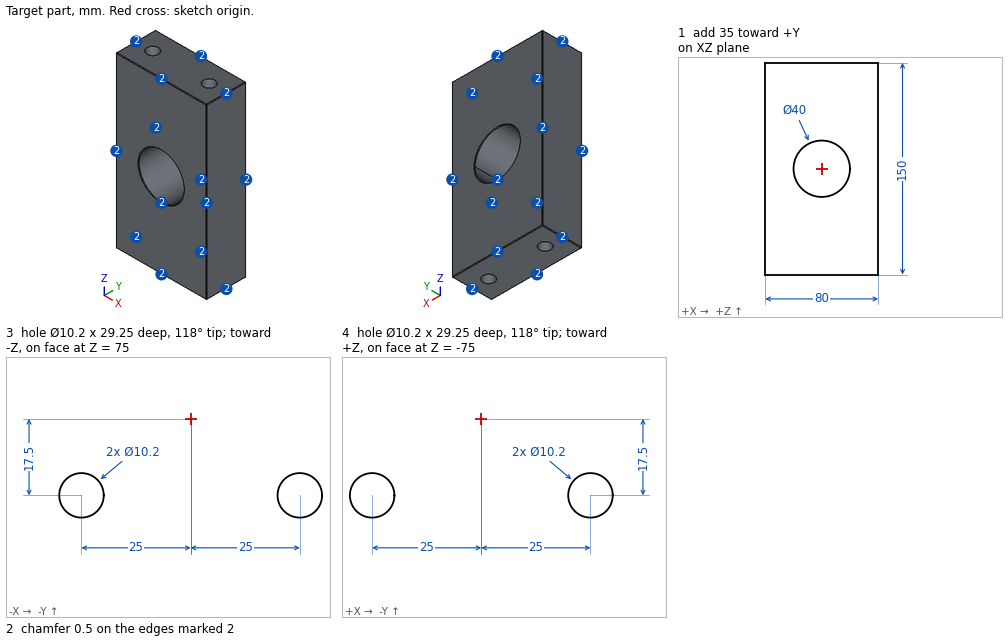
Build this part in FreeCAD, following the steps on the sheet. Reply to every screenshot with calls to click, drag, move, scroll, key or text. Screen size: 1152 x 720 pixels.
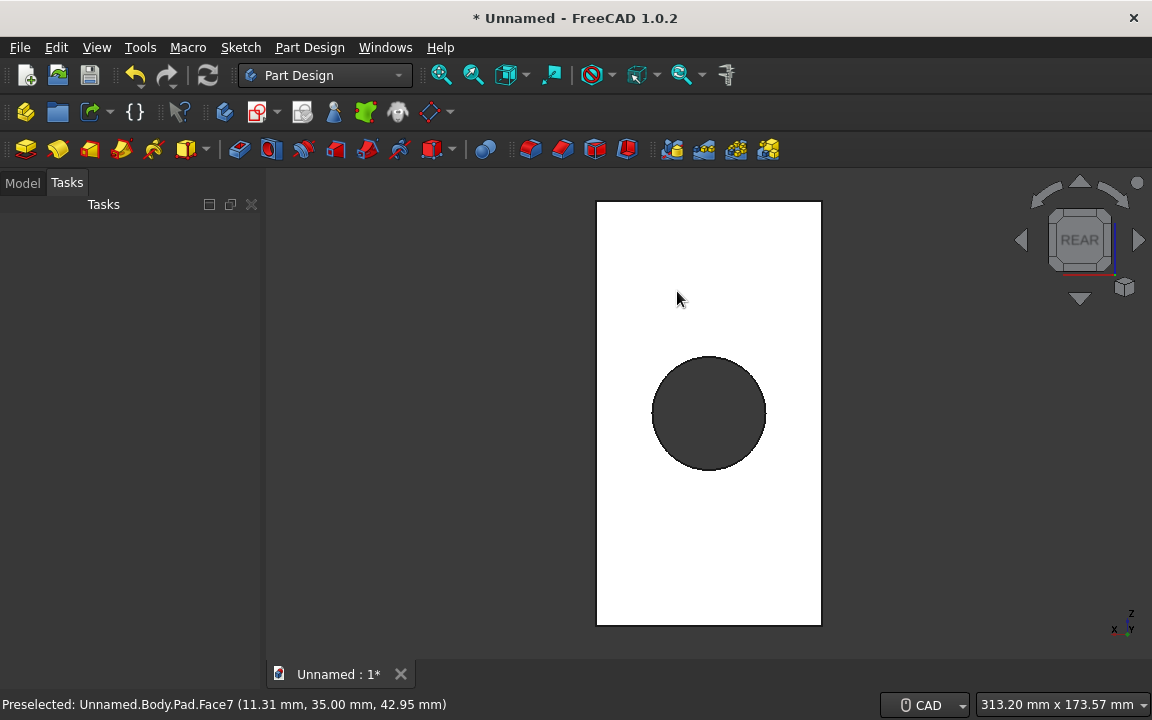
click(564, 150)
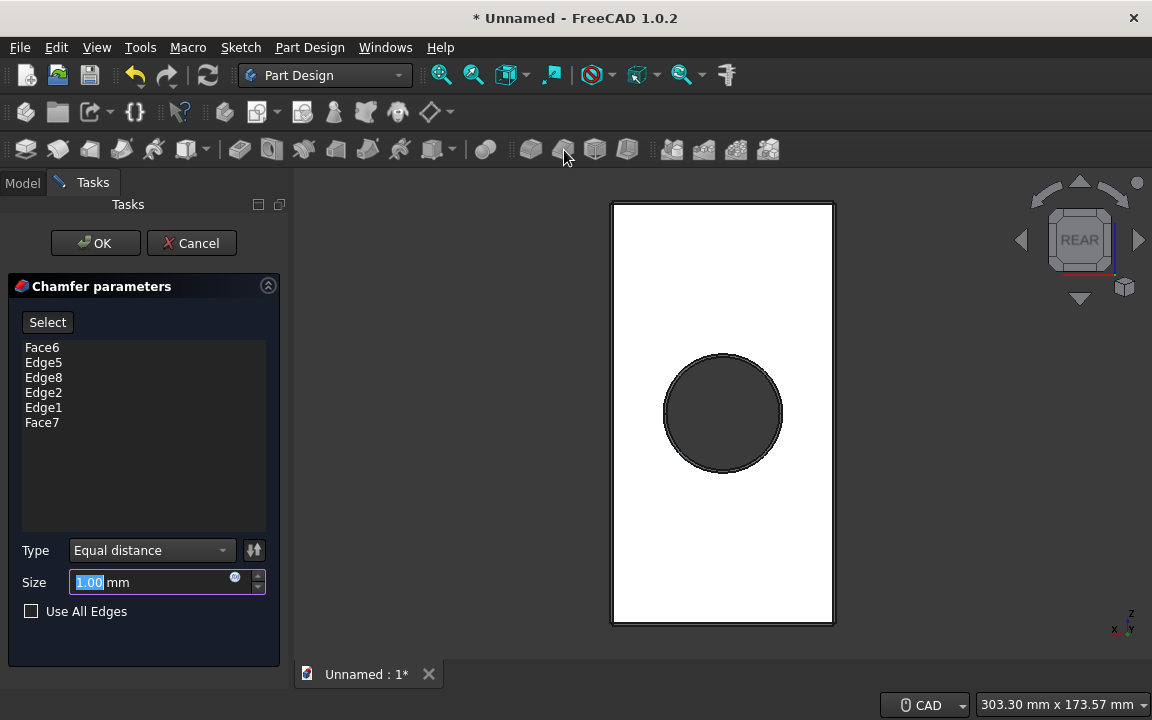
text(0.5)
key(Tab)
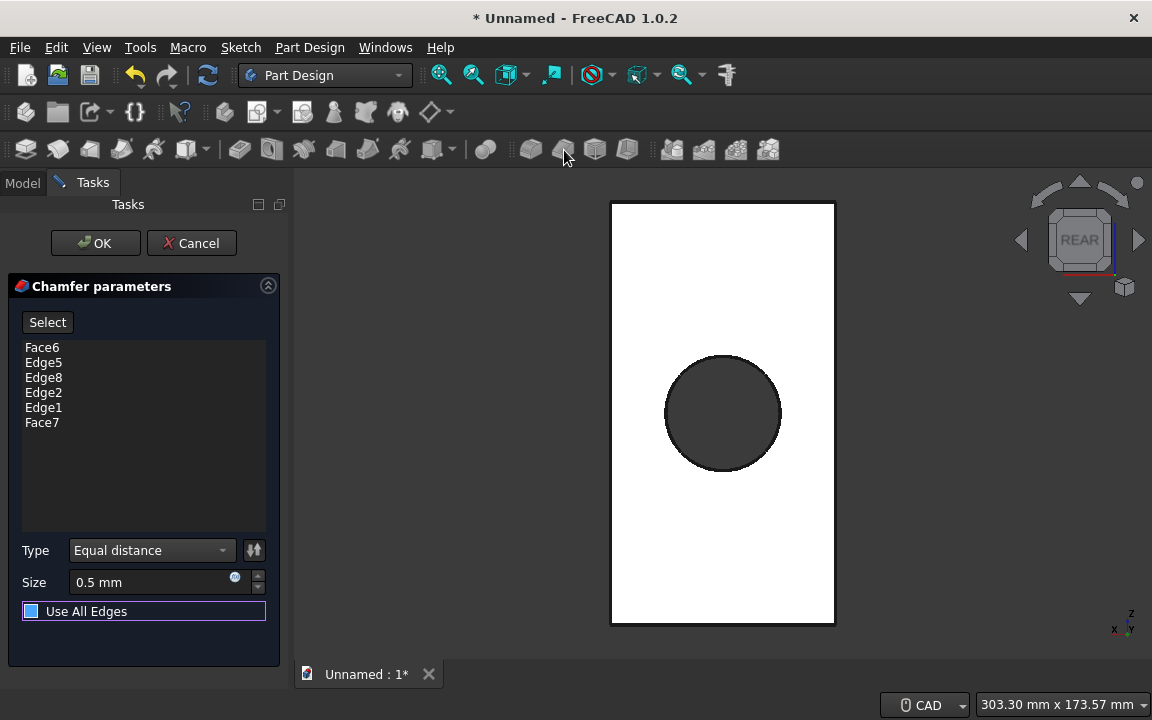
click(96, 243)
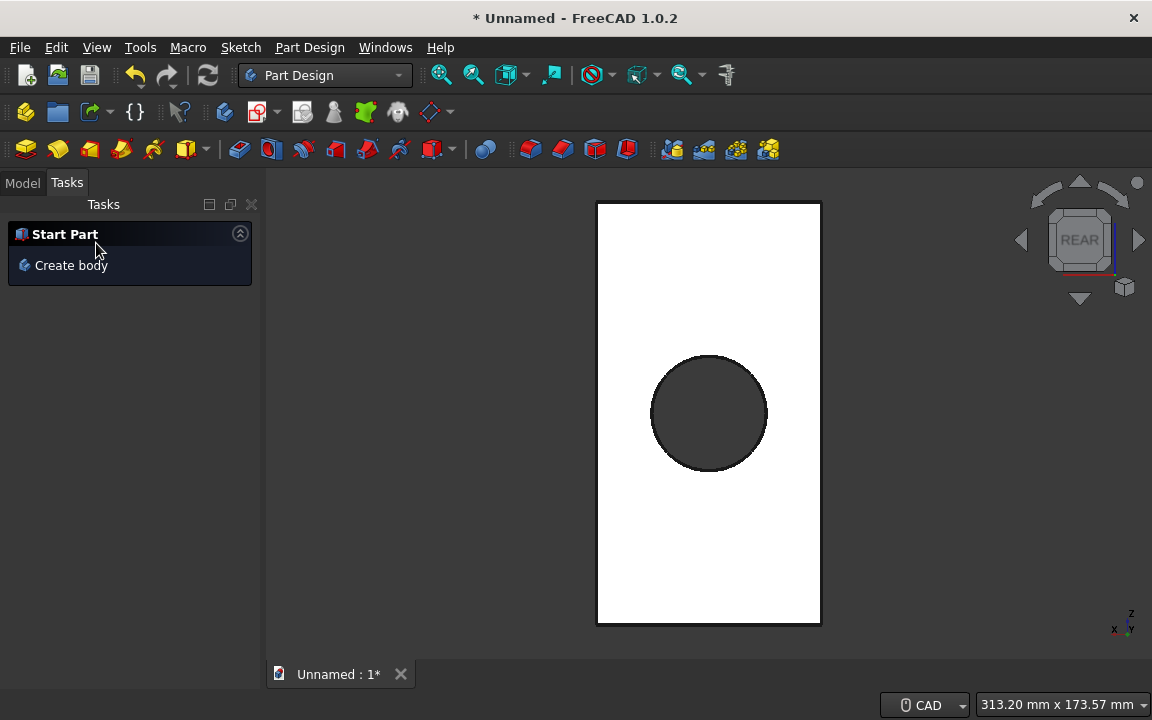
key(0)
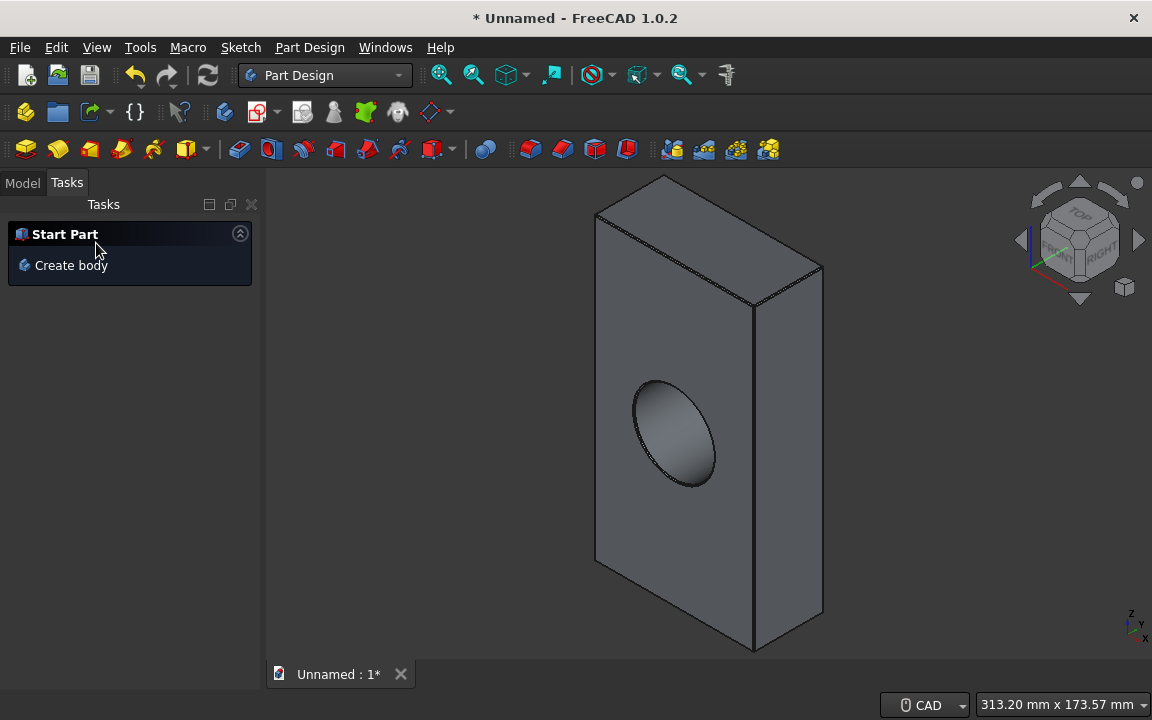
click(732, 252)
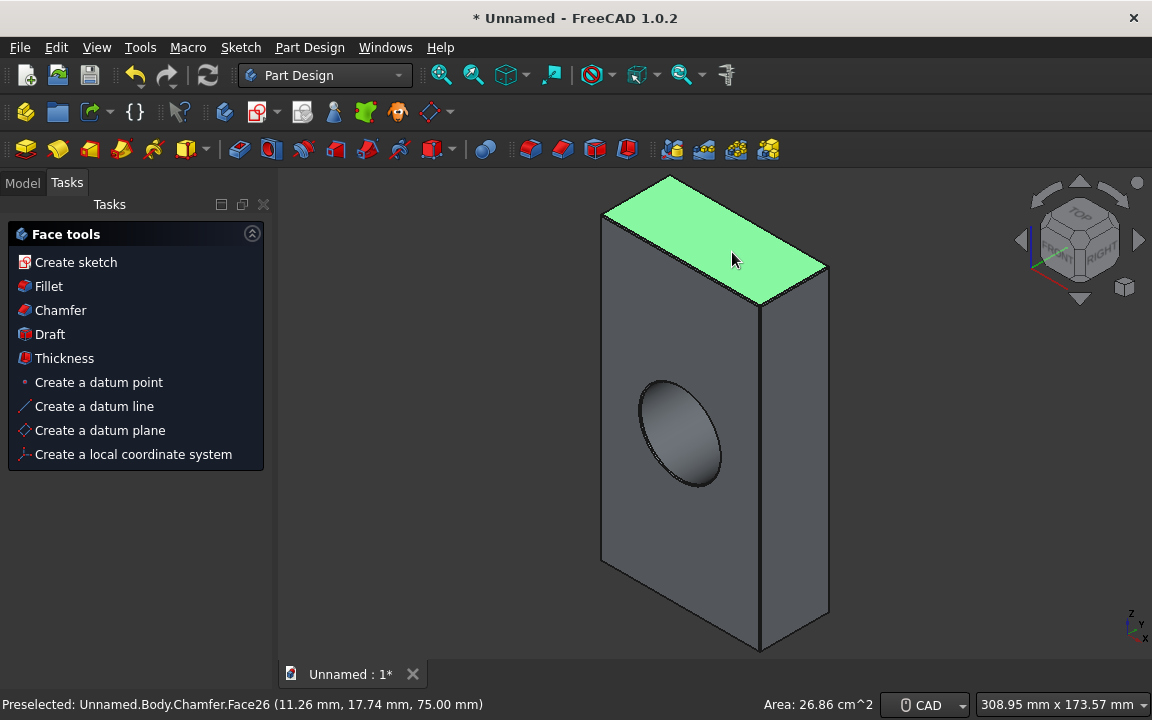
click(258, 112)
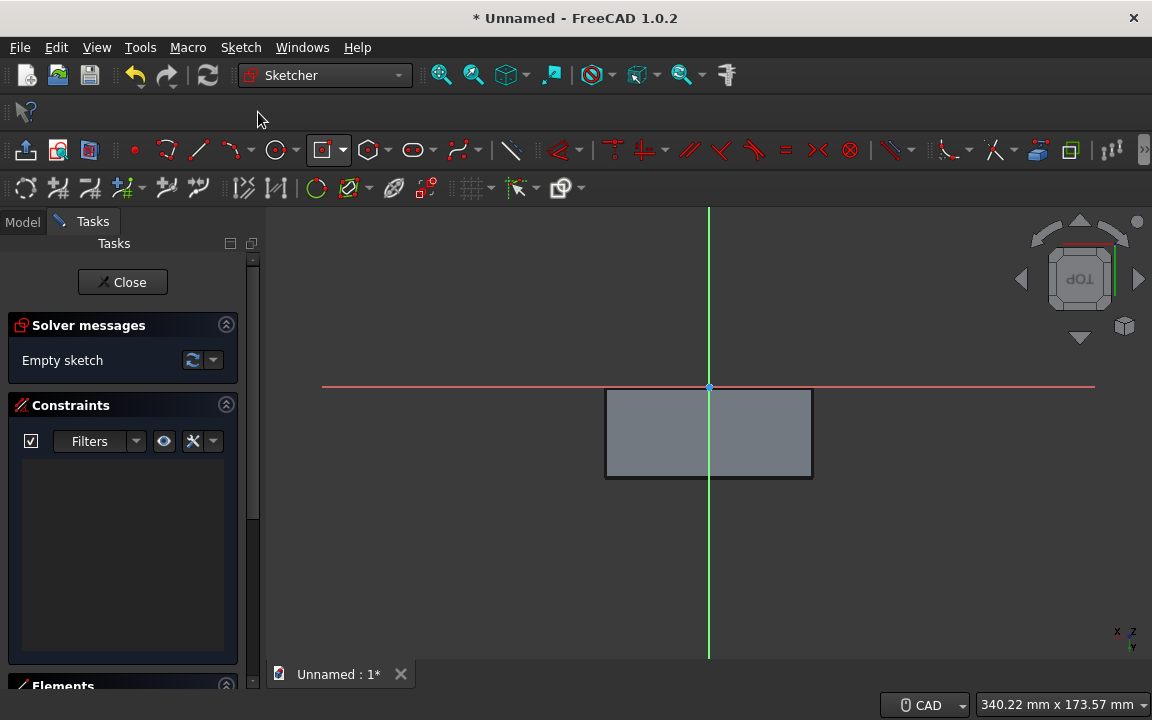
scroll(739, 410, up, 6)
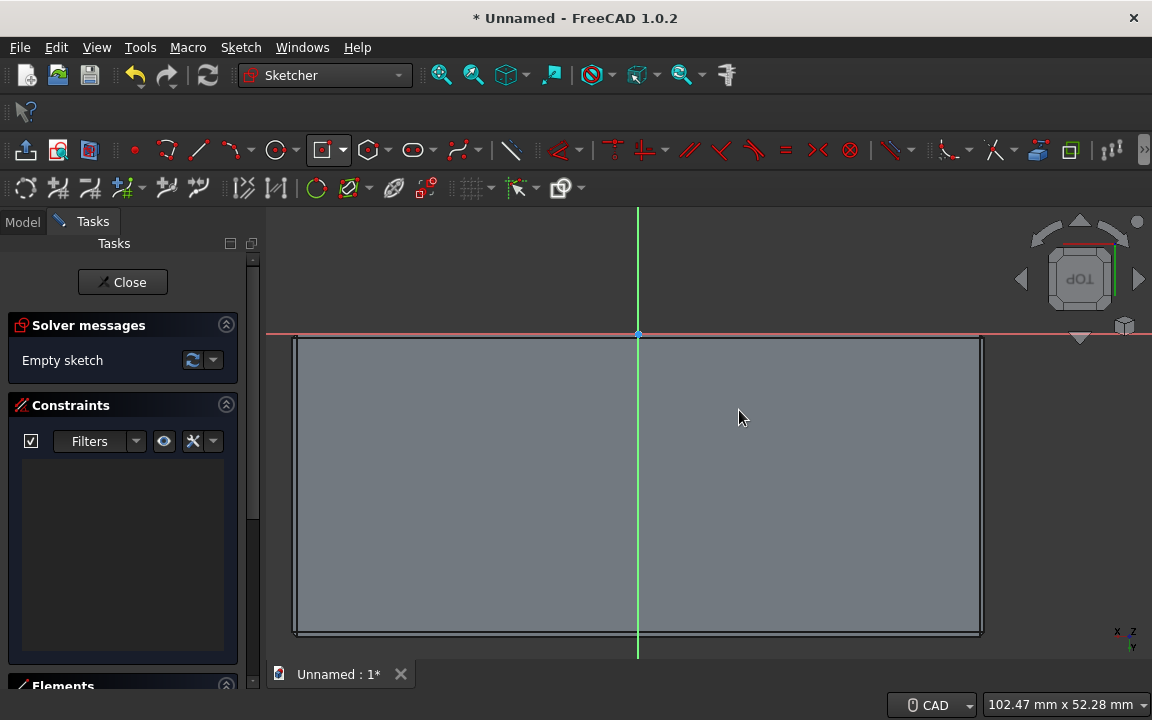
key(g)
key(c)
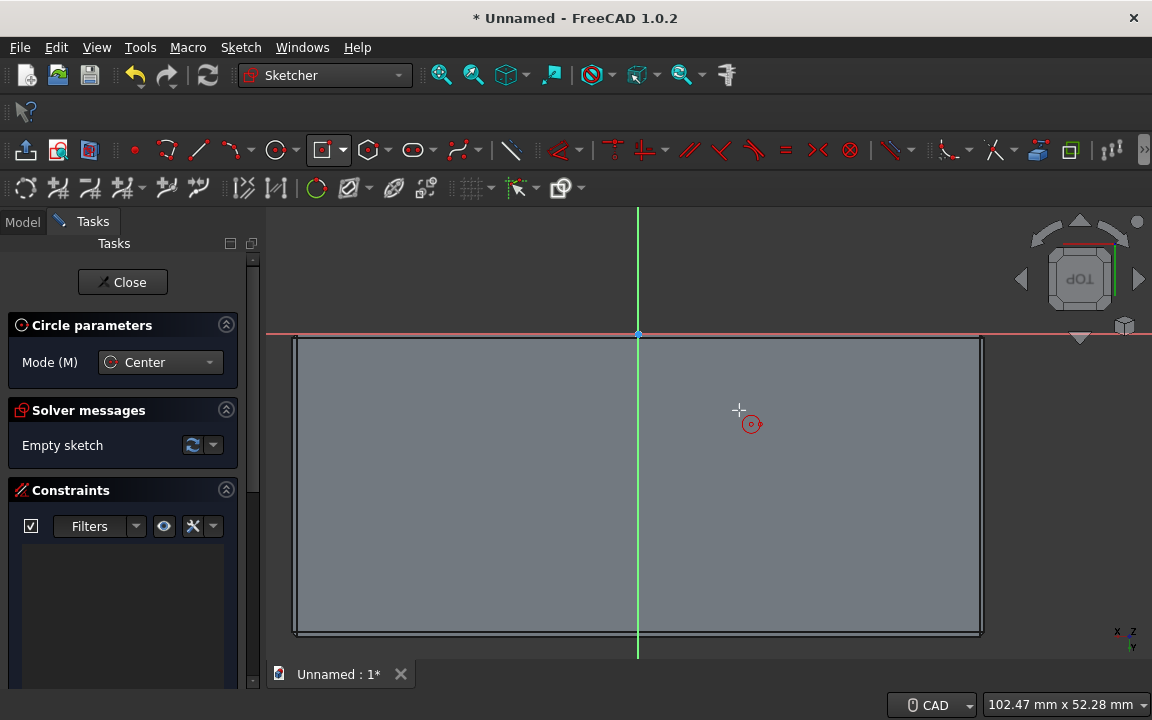
click(422, 485)
click(453, 454)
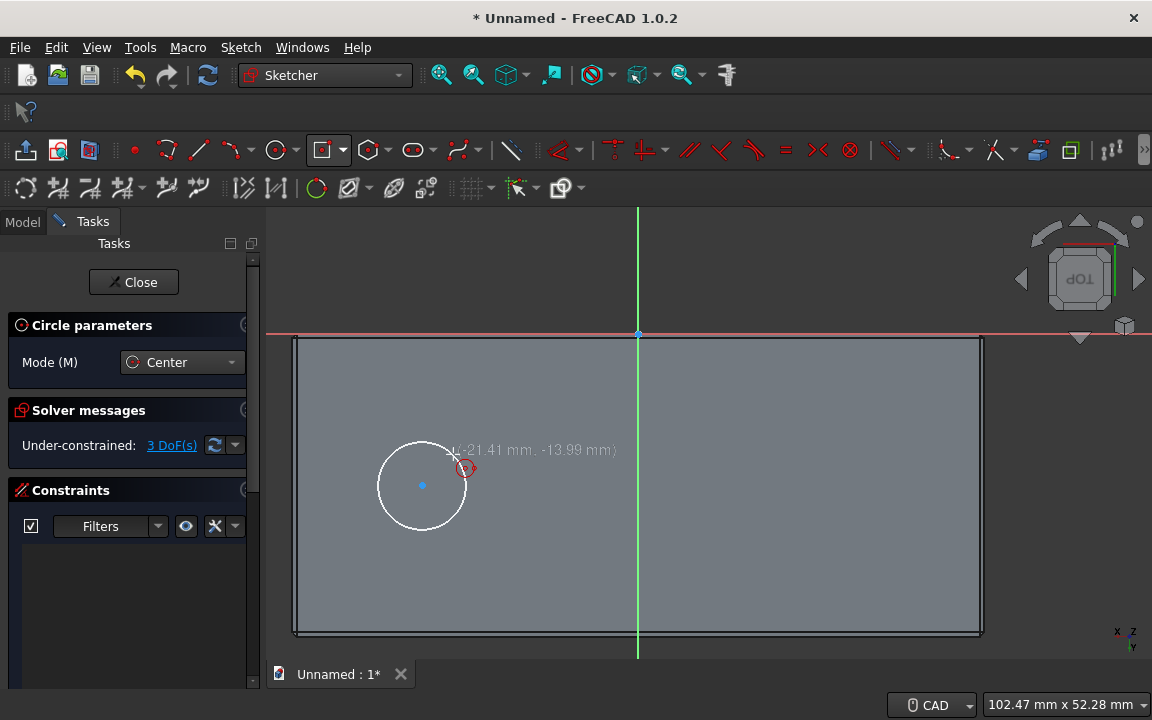
click(854, 485)
click(885, 454)
key(Escape)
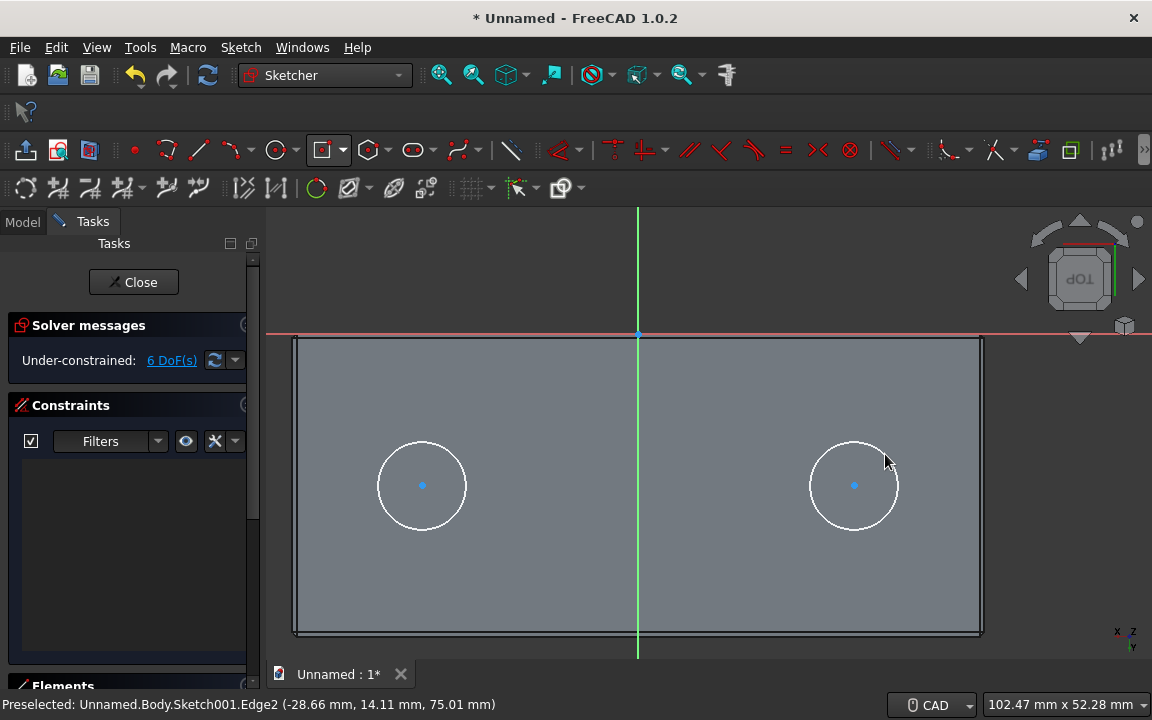
click(453, 455)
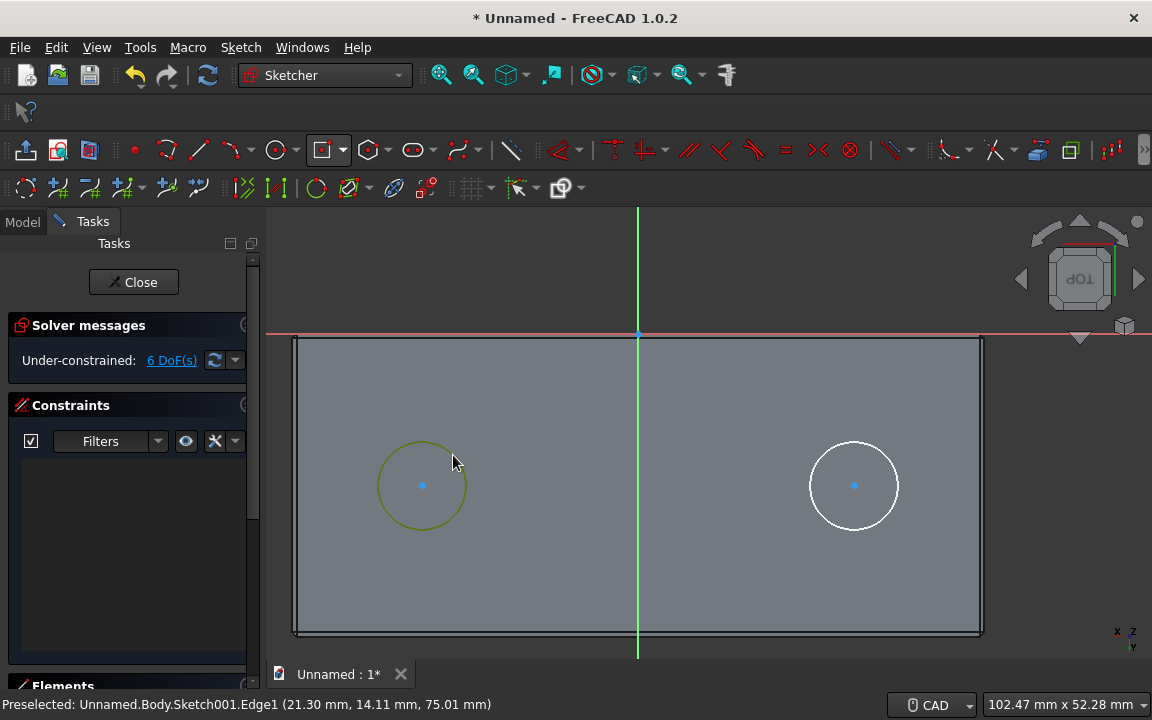
click(885, 455)